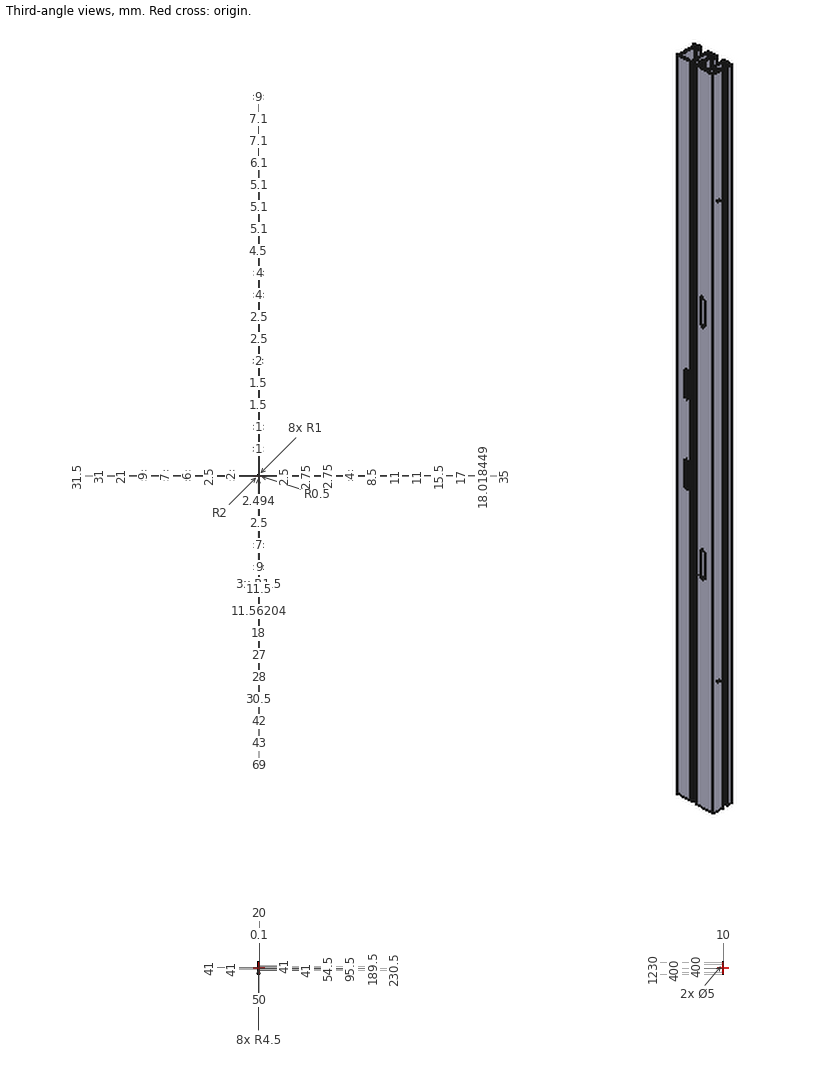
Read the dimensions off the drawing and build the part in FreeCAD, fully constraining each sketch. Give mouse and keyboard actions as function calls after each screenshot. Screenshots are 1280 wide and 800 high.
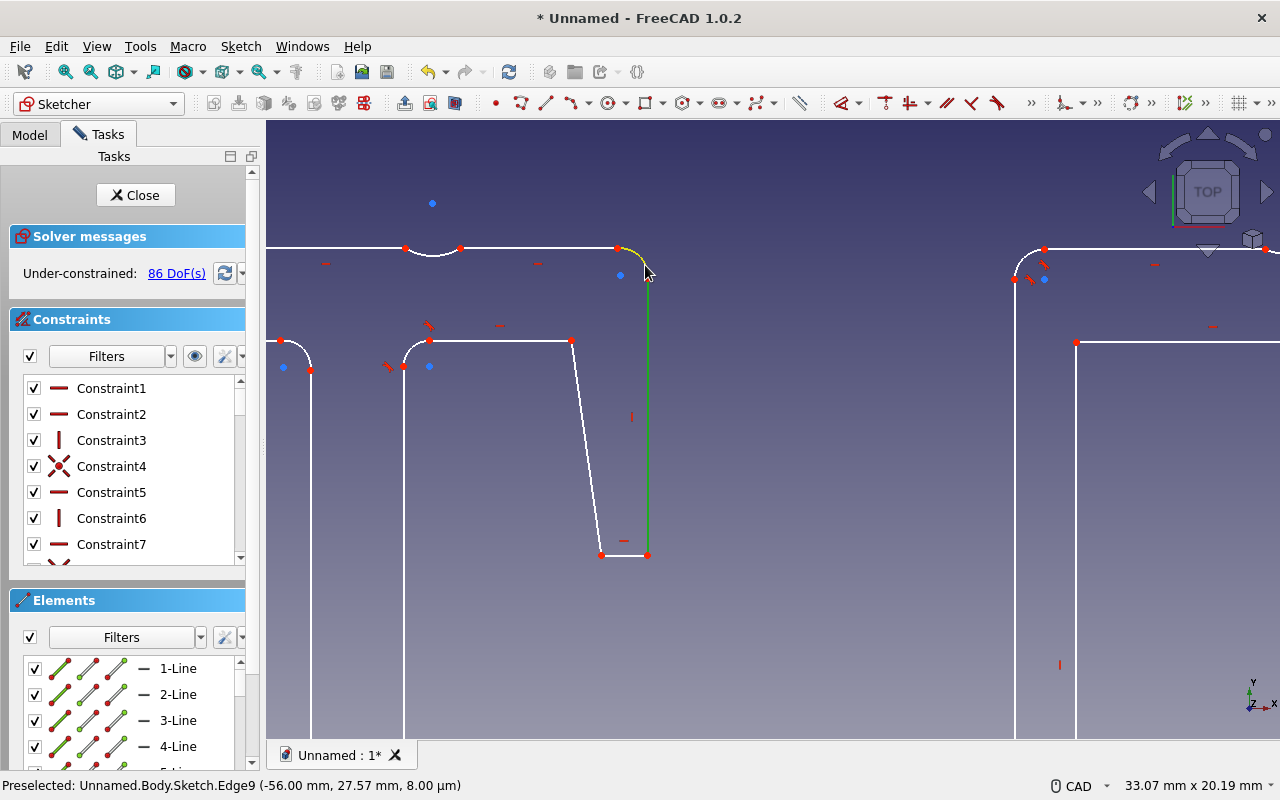
click(645, 264)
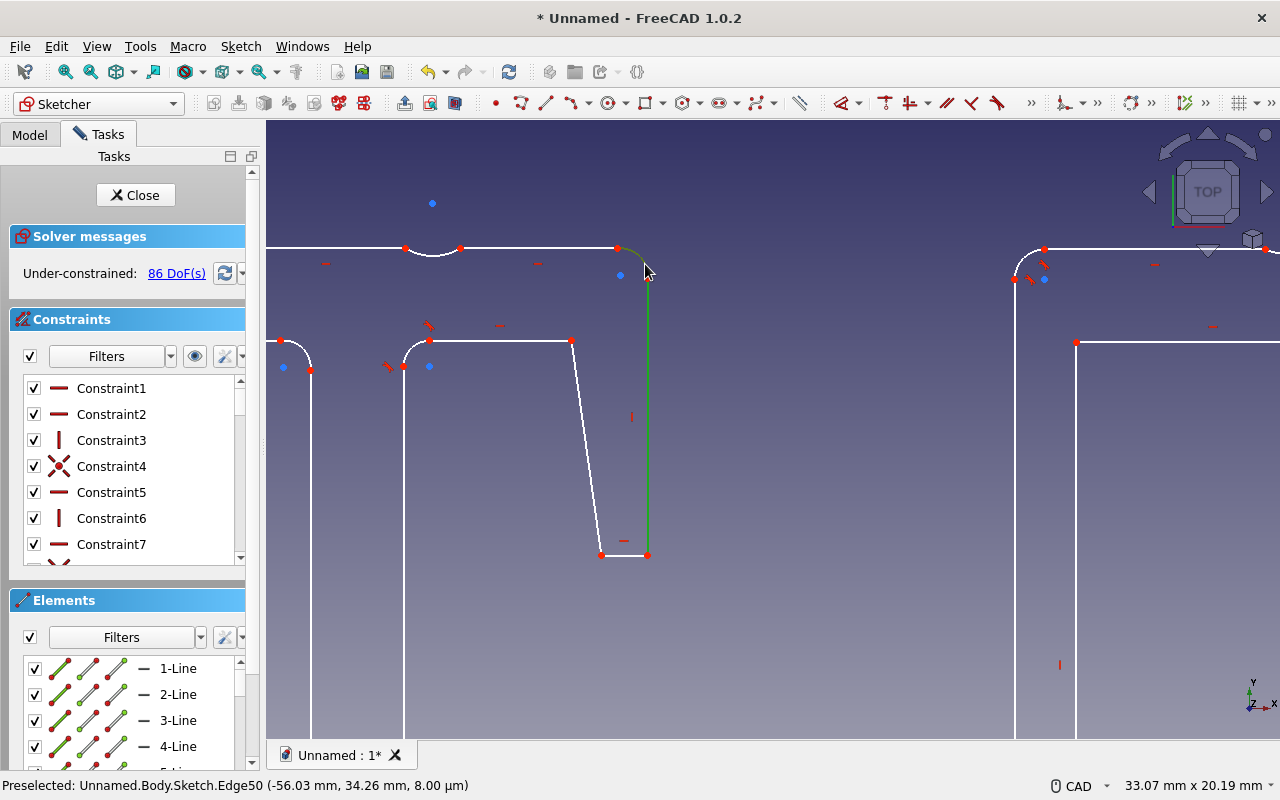
click(997, 104)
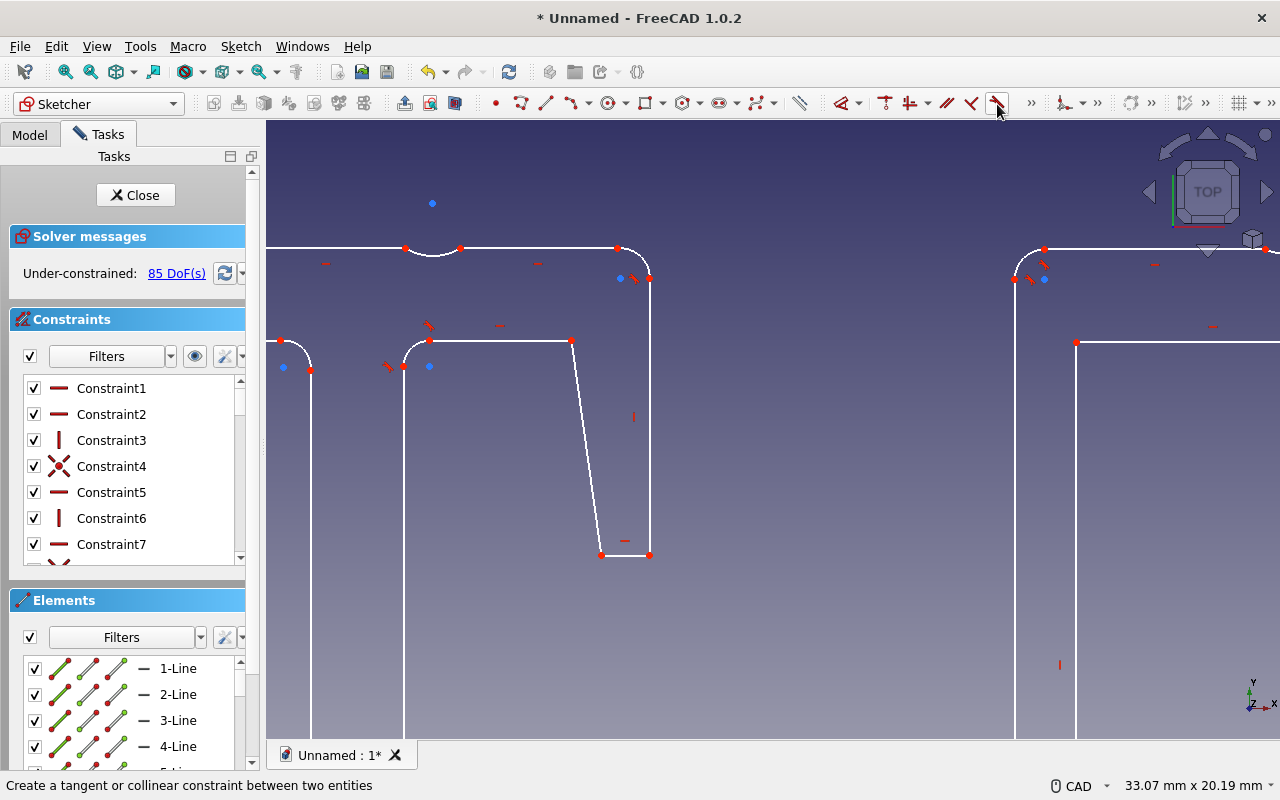
scroll(512, 314, down, 7)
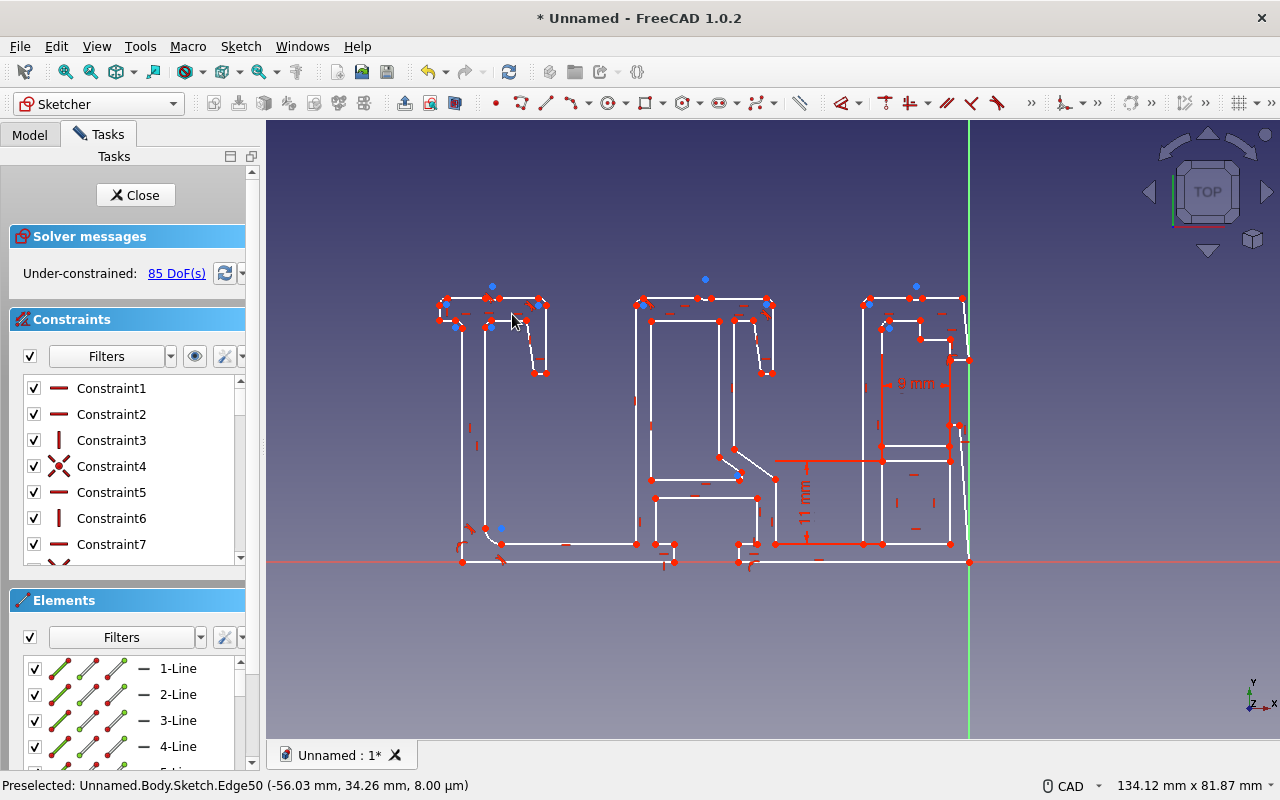
click(527, 298)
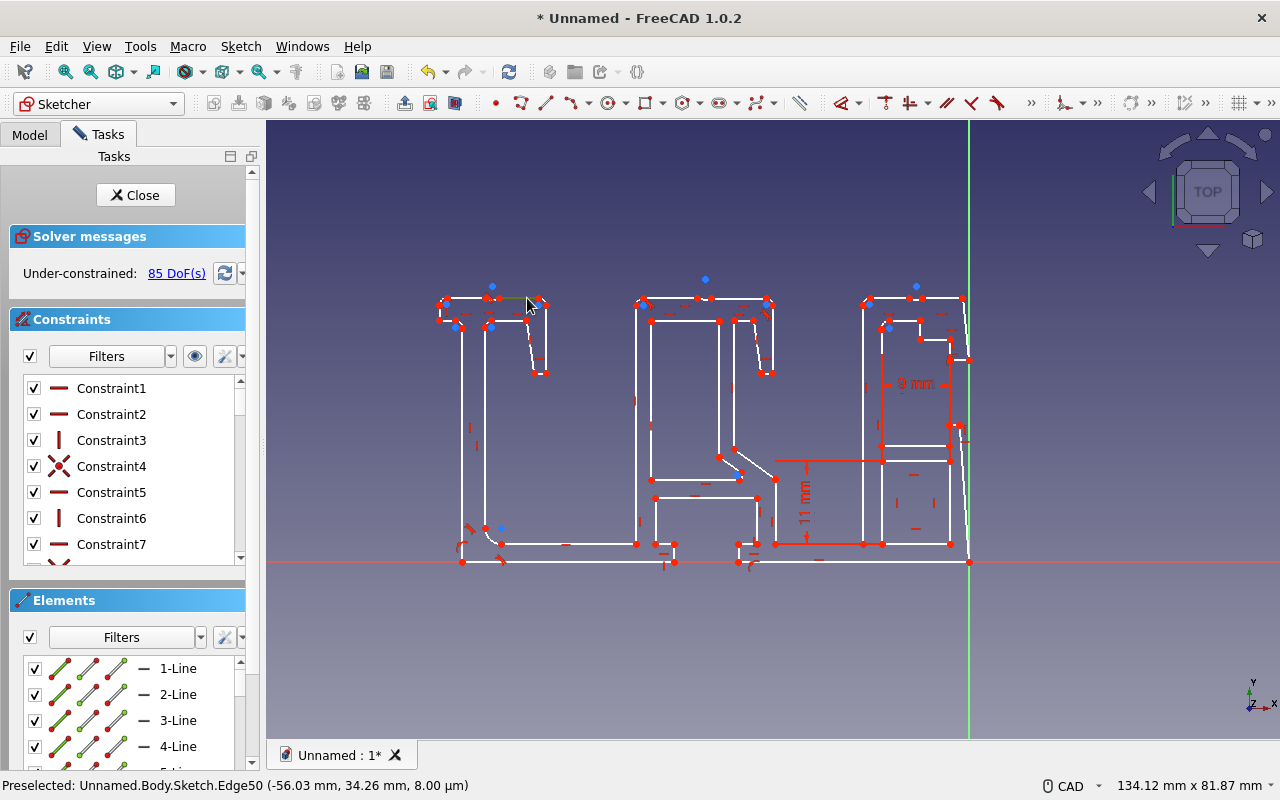
scroll(544, 300, up, 5)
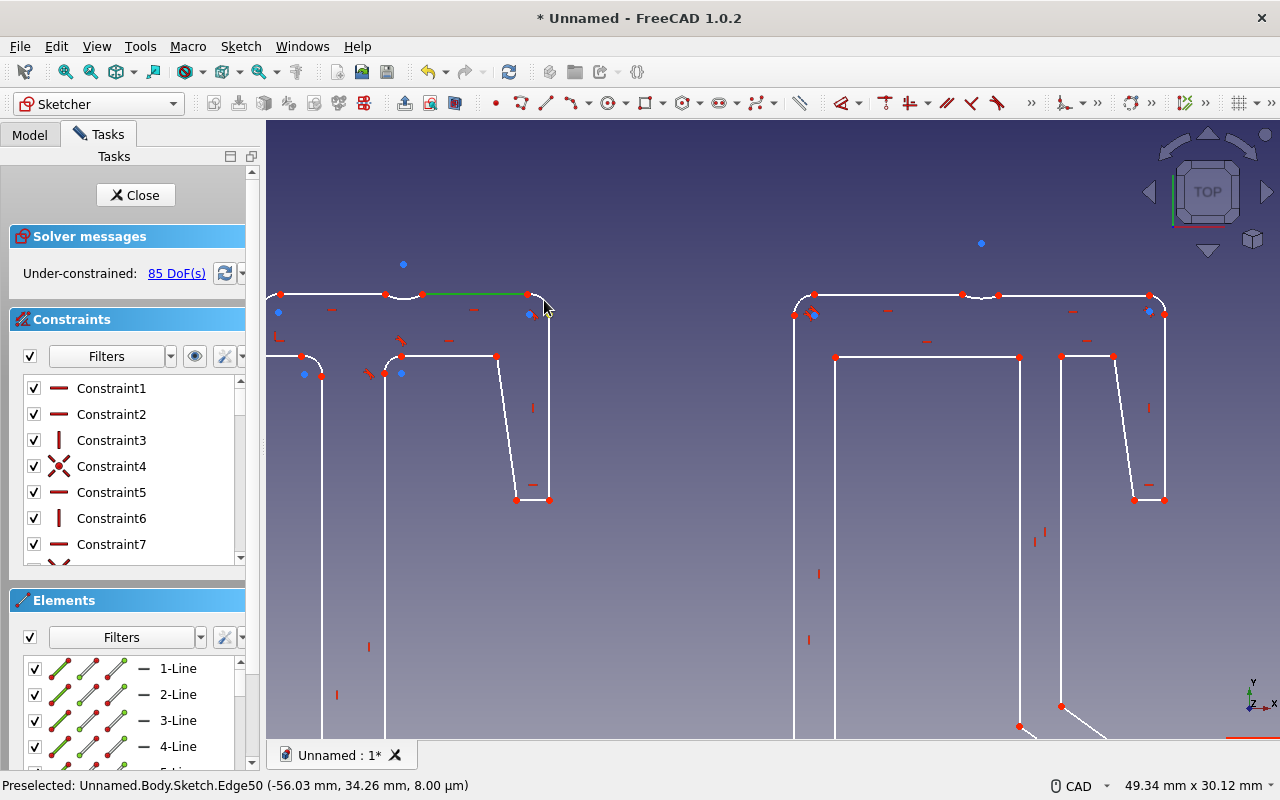
click(543, 299)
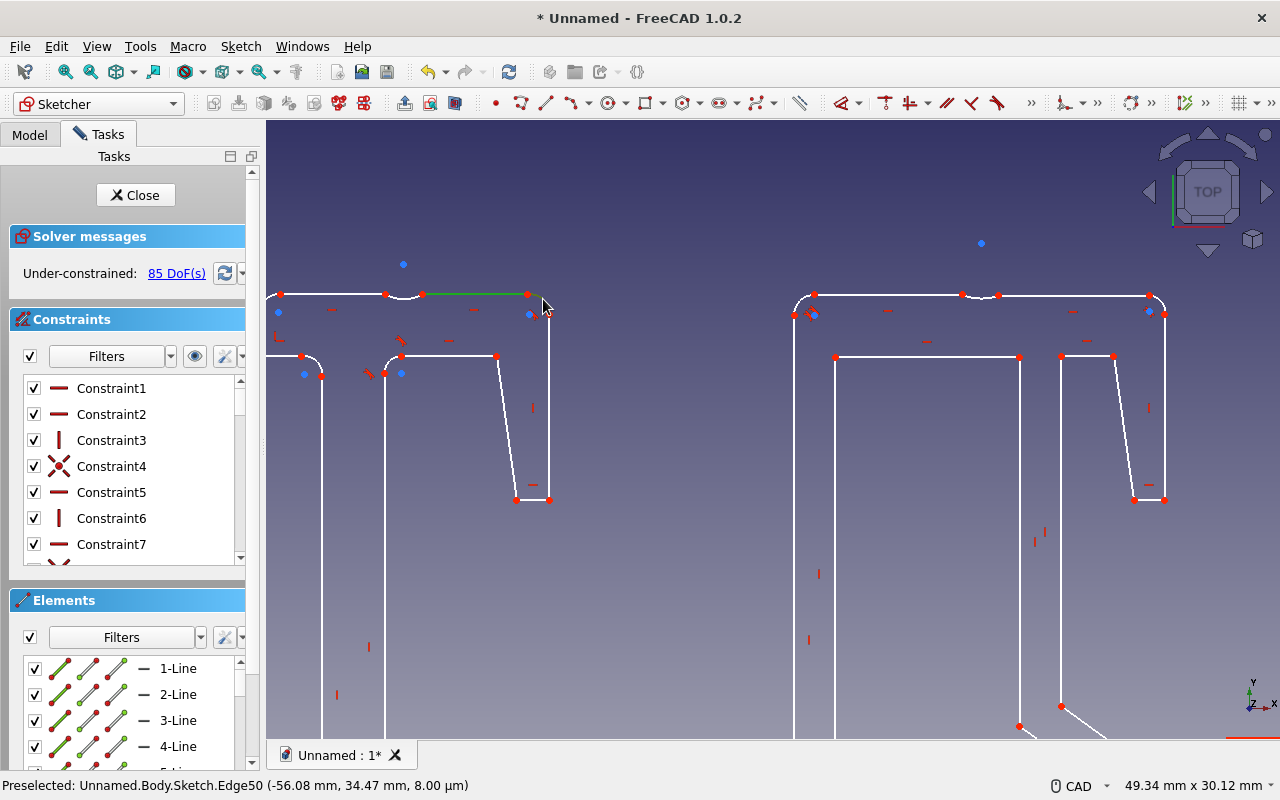
click(997, 104)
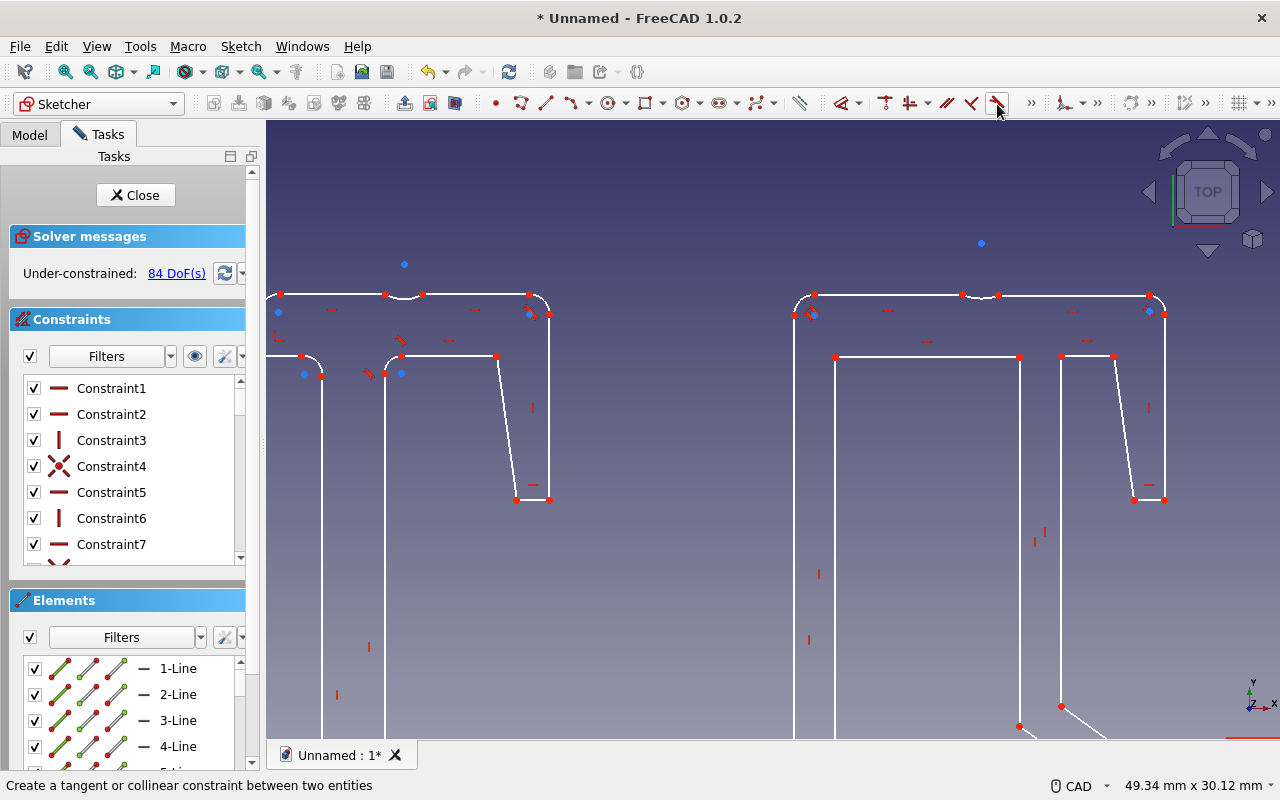
click(354, 294)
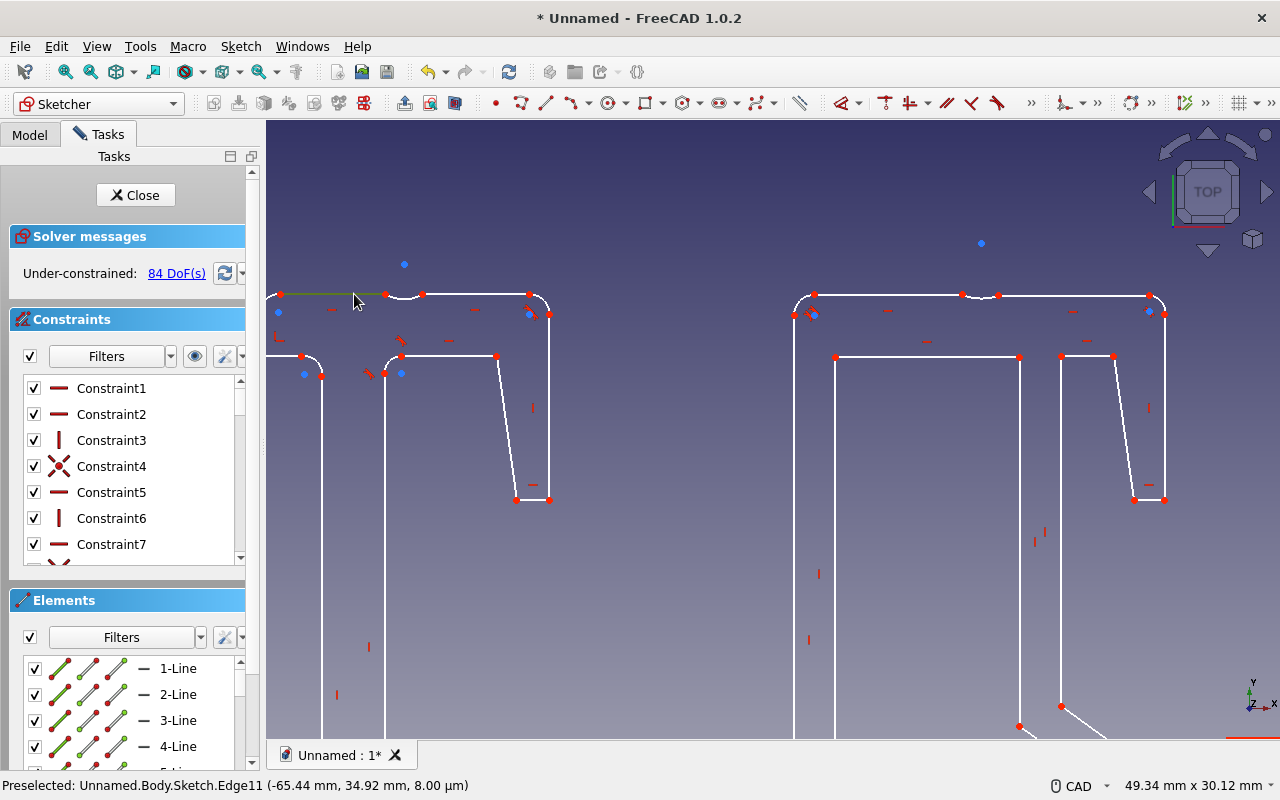
scroll(544, 300, down, 5)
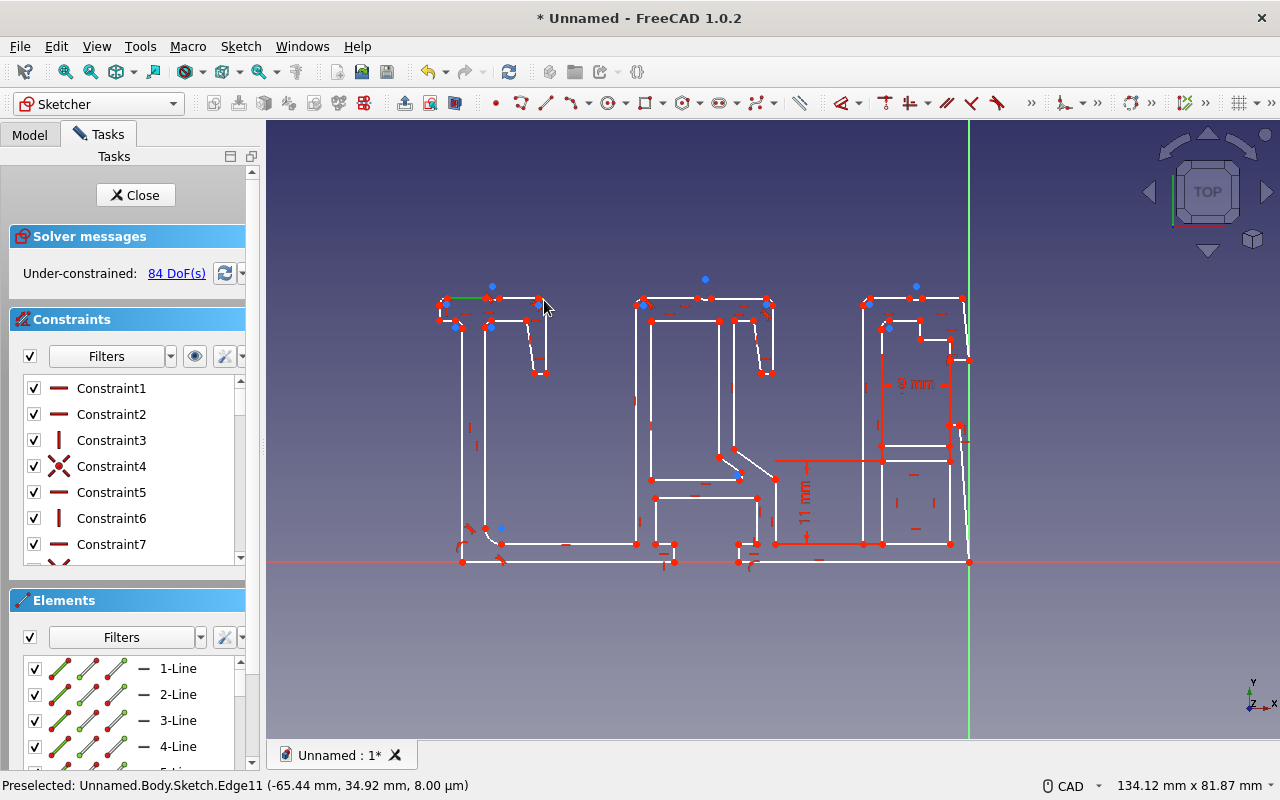
scroll(444, 299, up, 7)